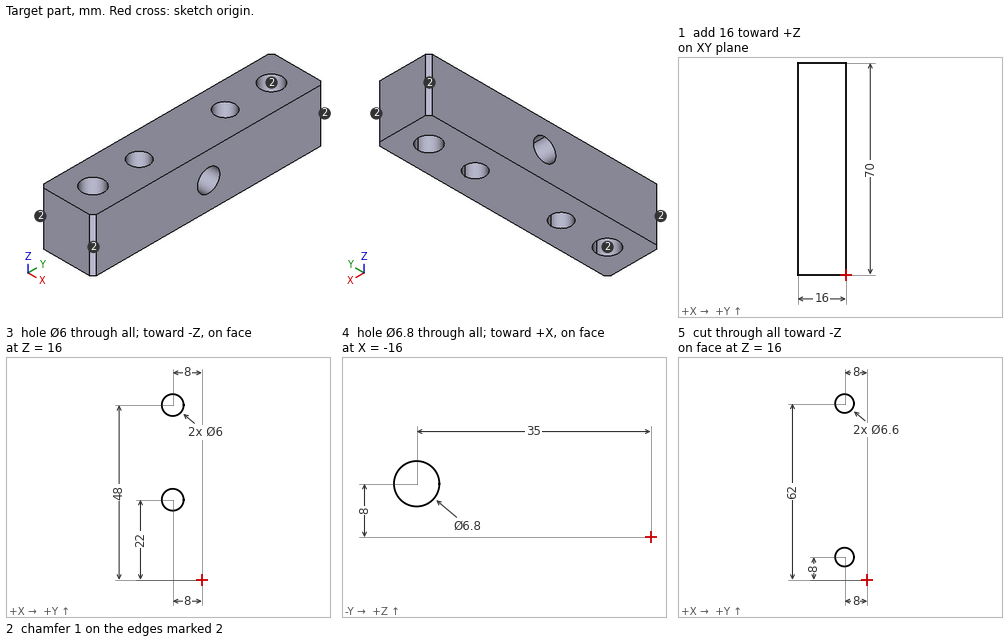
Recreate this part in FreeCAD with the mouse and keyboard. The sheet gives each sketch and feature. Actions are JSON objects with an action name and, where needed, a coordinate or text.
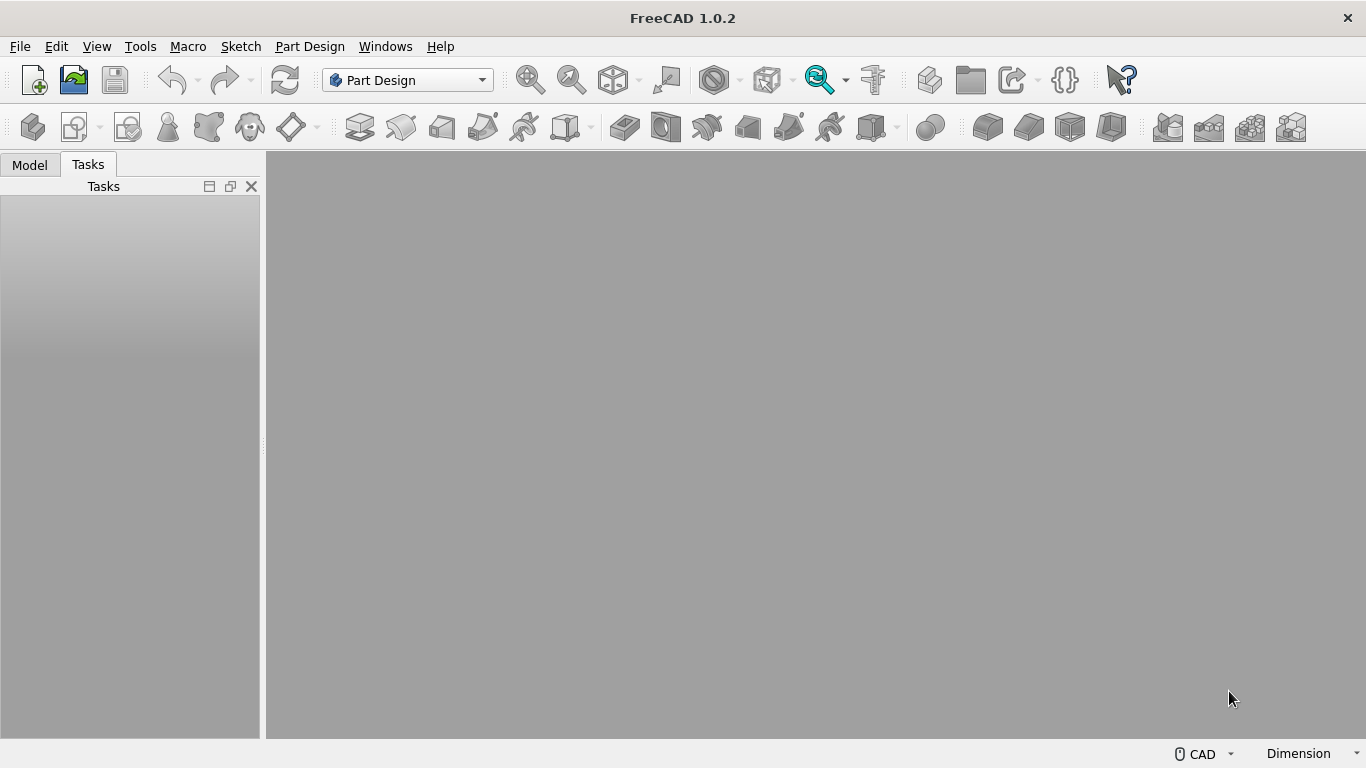
{"action": "key", "text": "ctrl+n"}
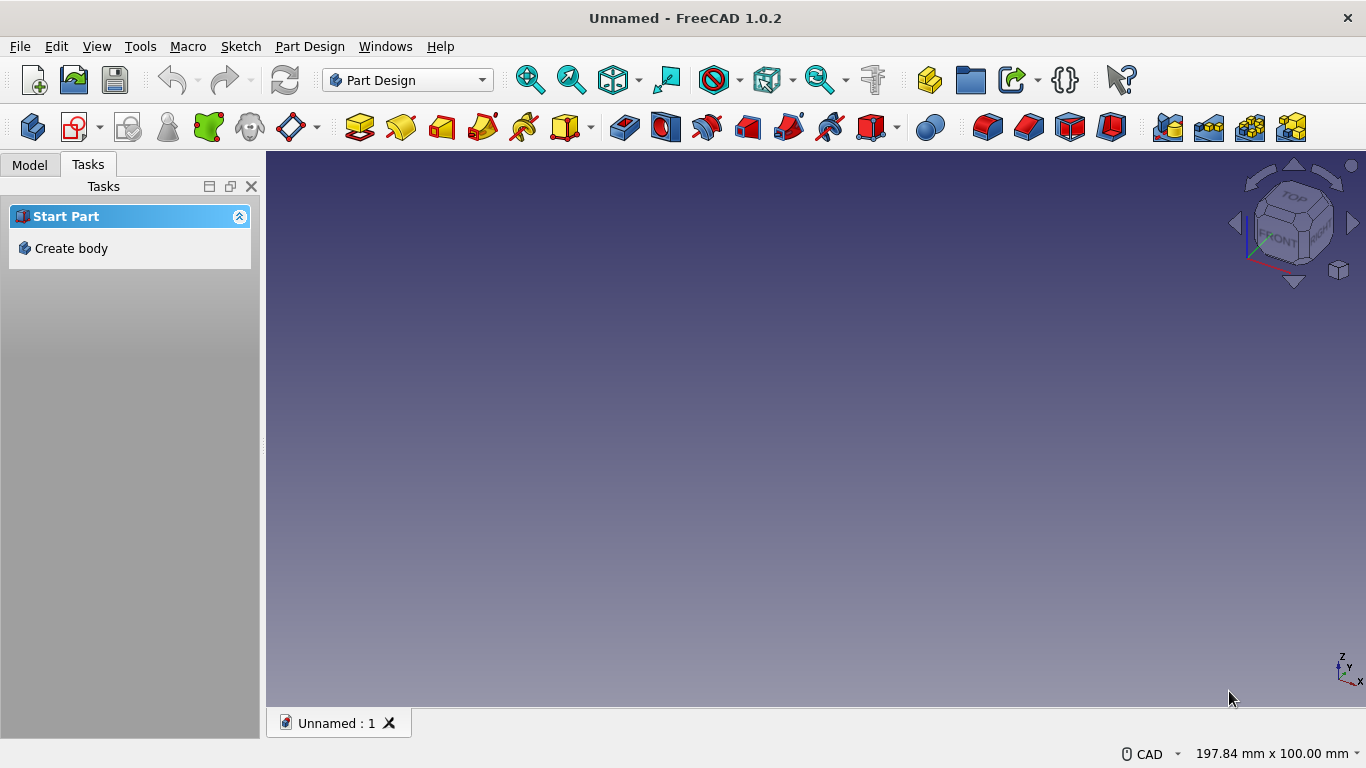
{"action": "left_click", "coordinate": [74, 128]}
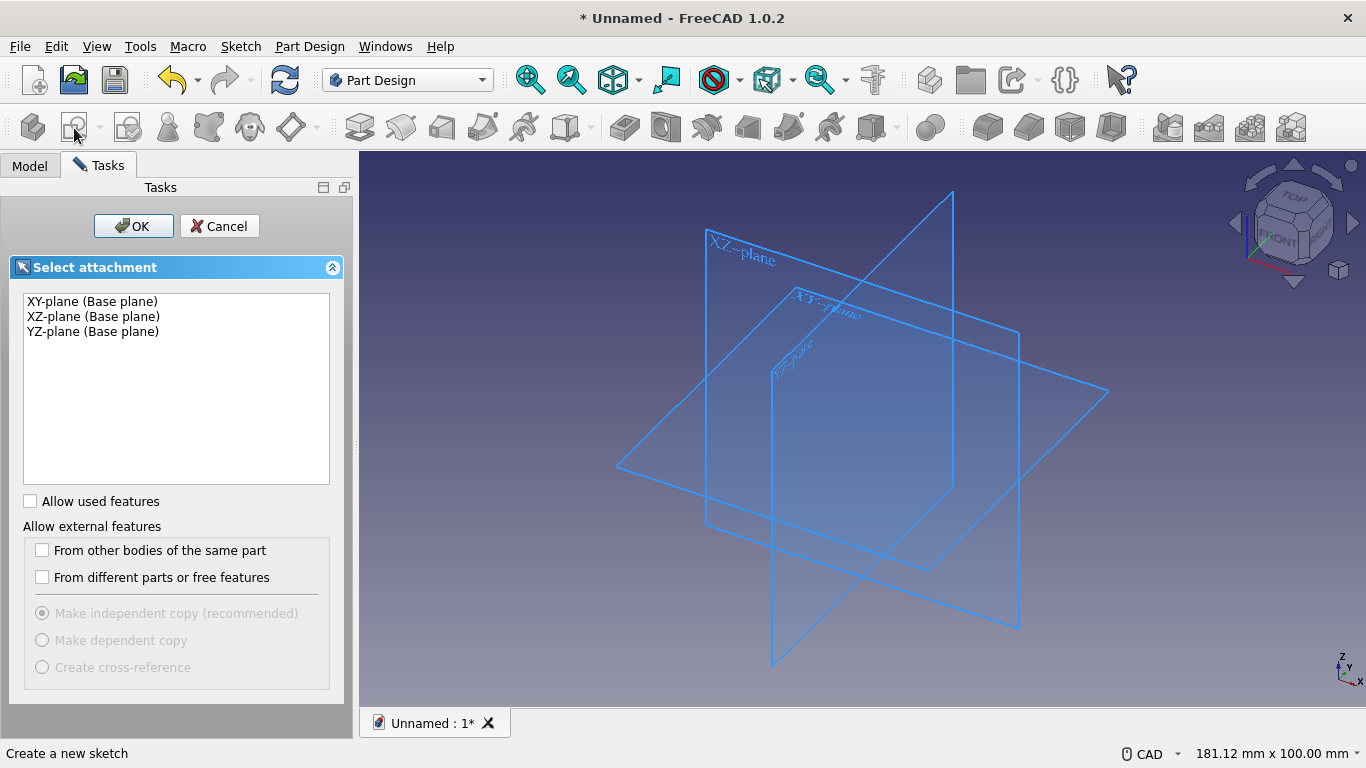
{"action": "left_click", "coordinate": [84, 302]}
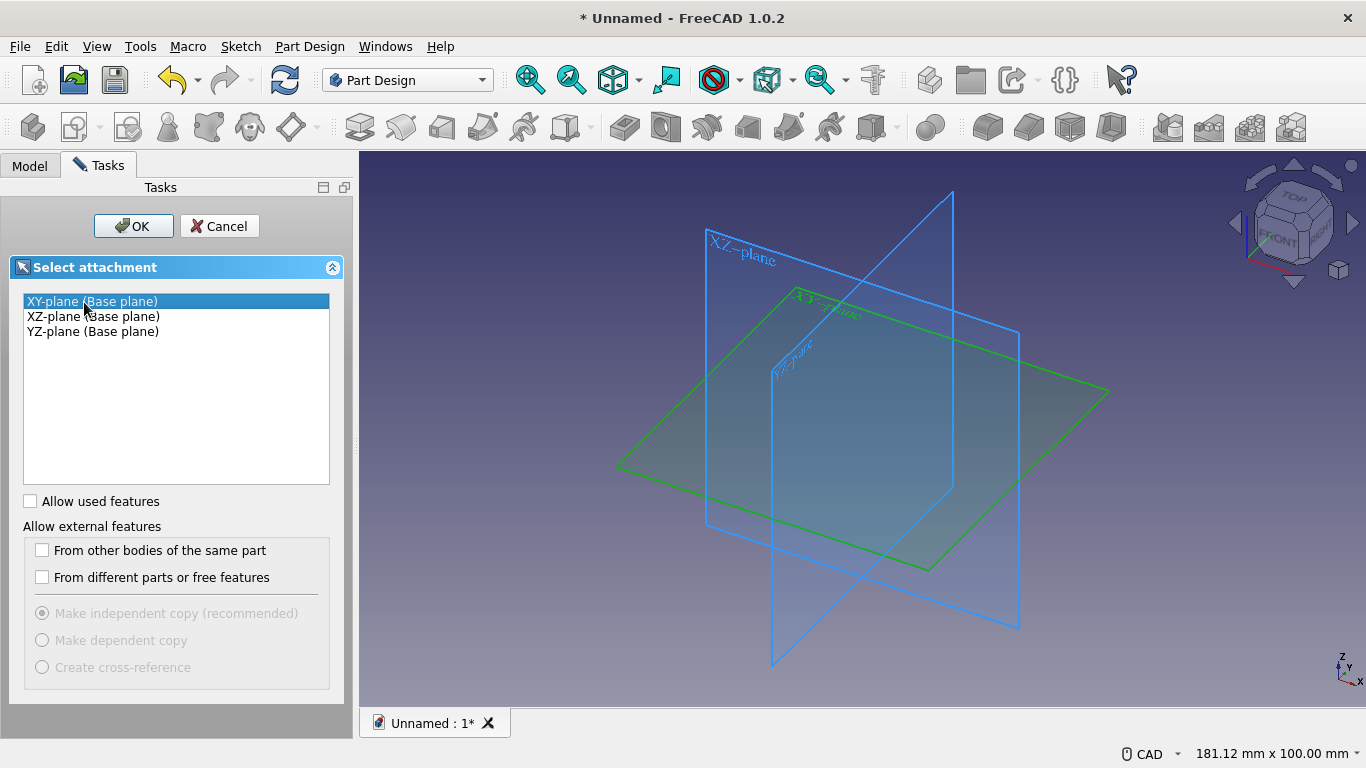
{"action": "left_click", "coordinate": [134, 226]}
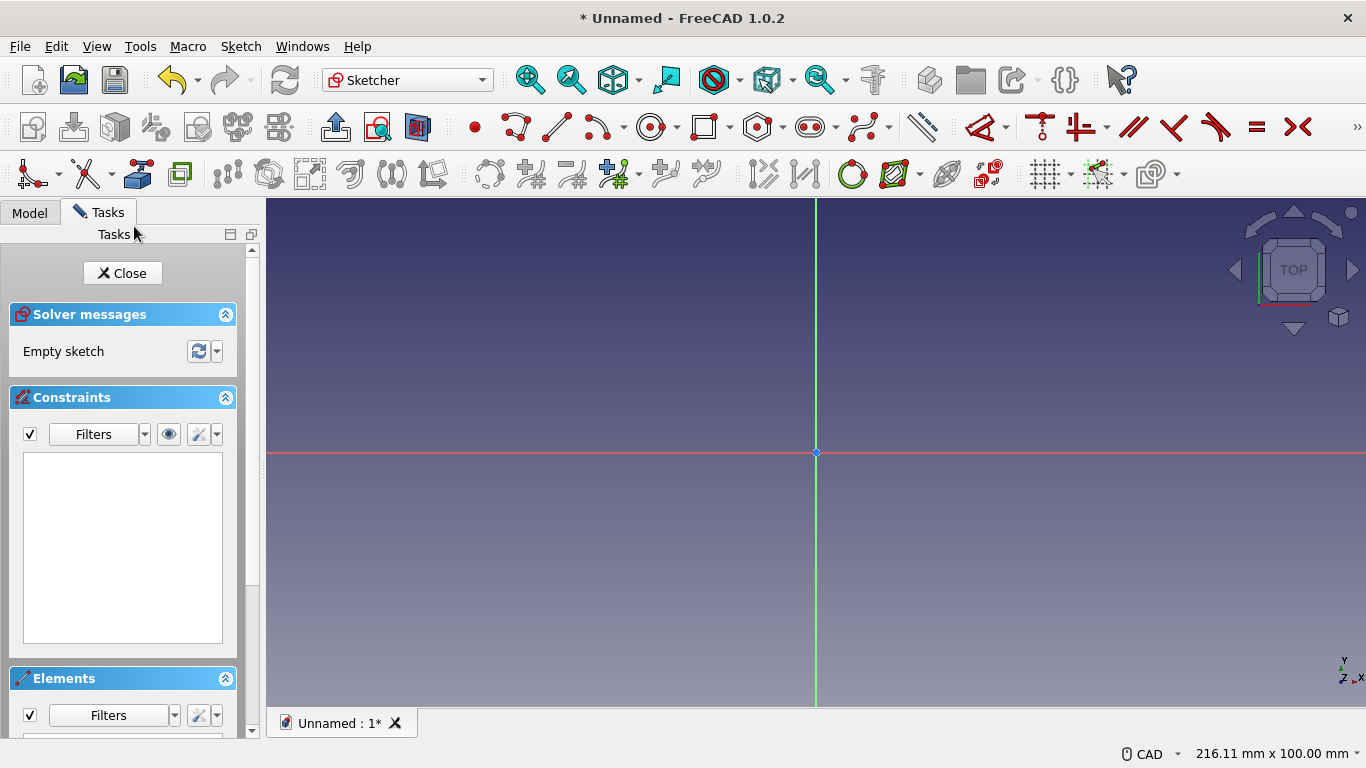
{"action": "scroll", "coordinate": [691, 679], "scroll_direction": "down", "scroll_amount": 2}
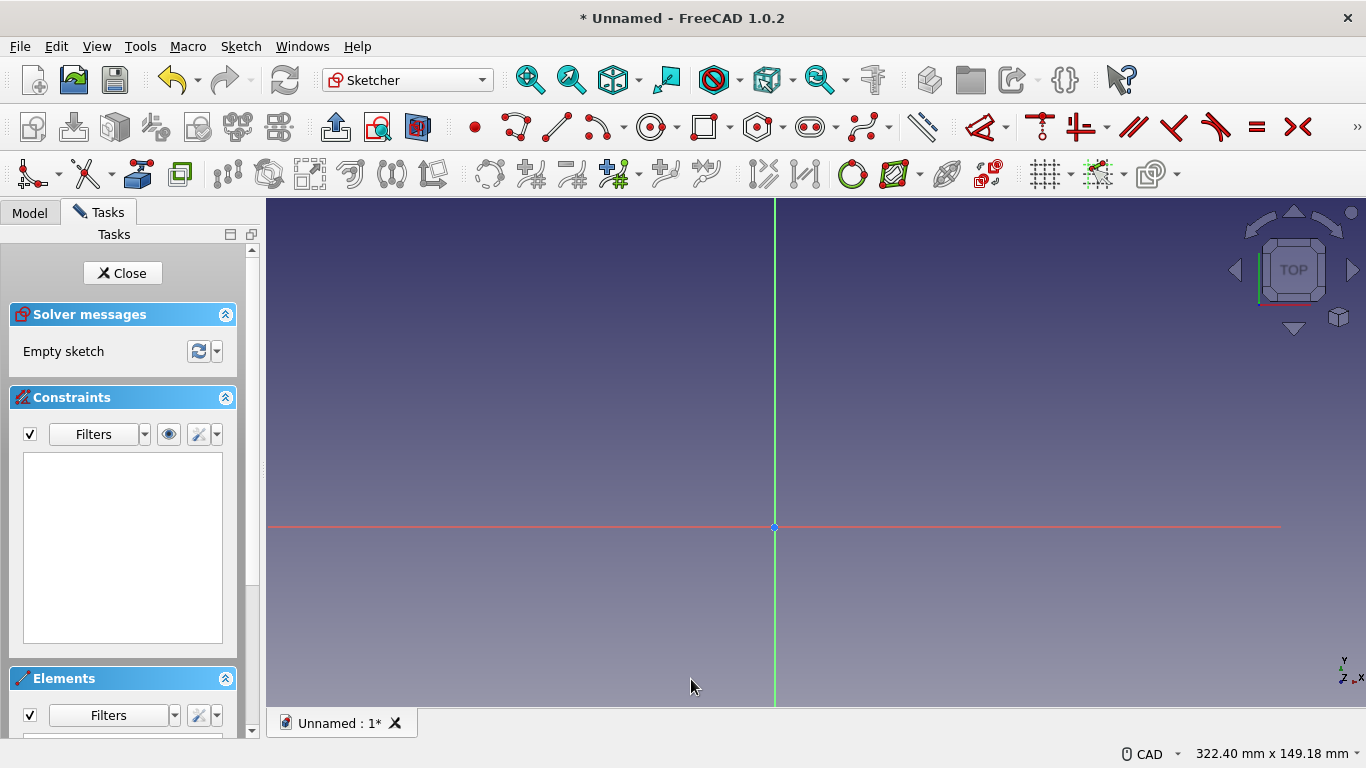
{"action": "left_click", "coordinate": [704, 128]}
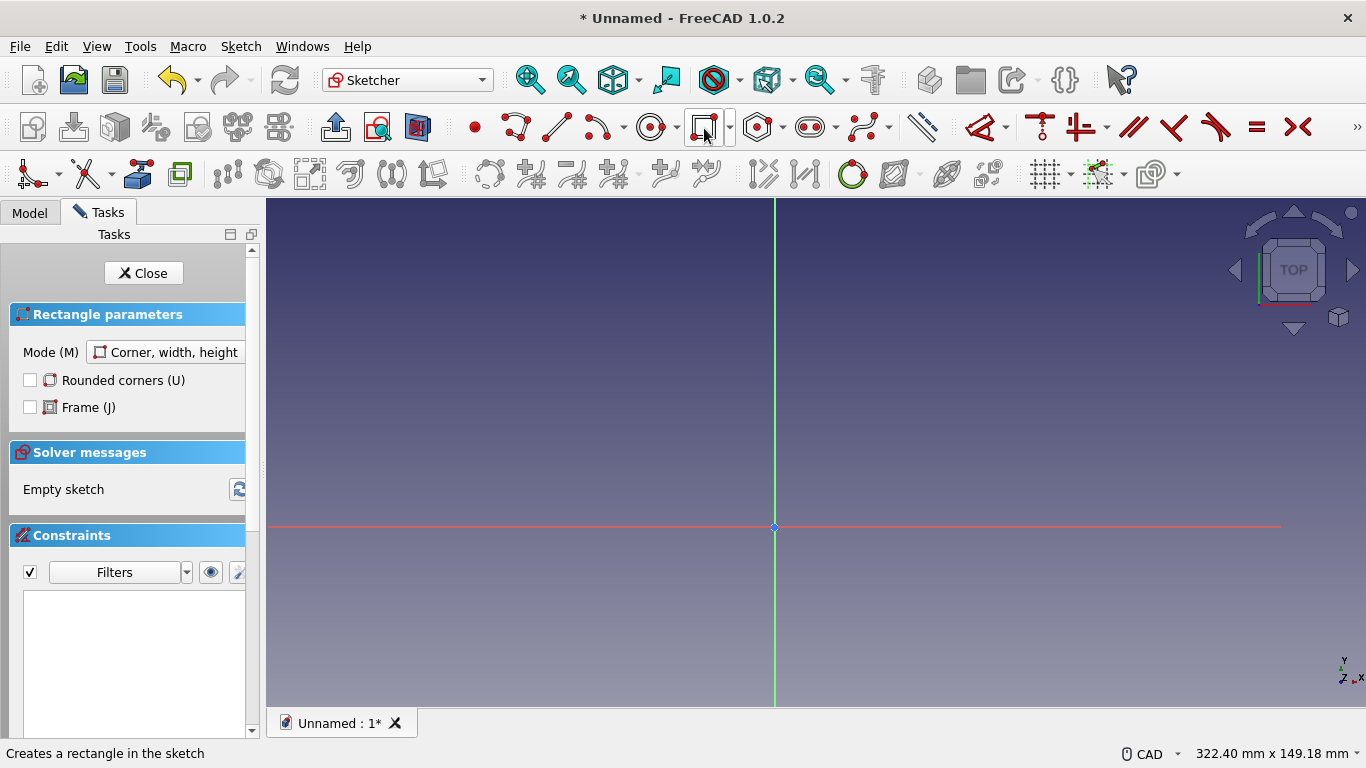
{"action": "left_click", "coordinate": [775, 527]}
{"action": "mouse_move", "coordinate": [720, 289]}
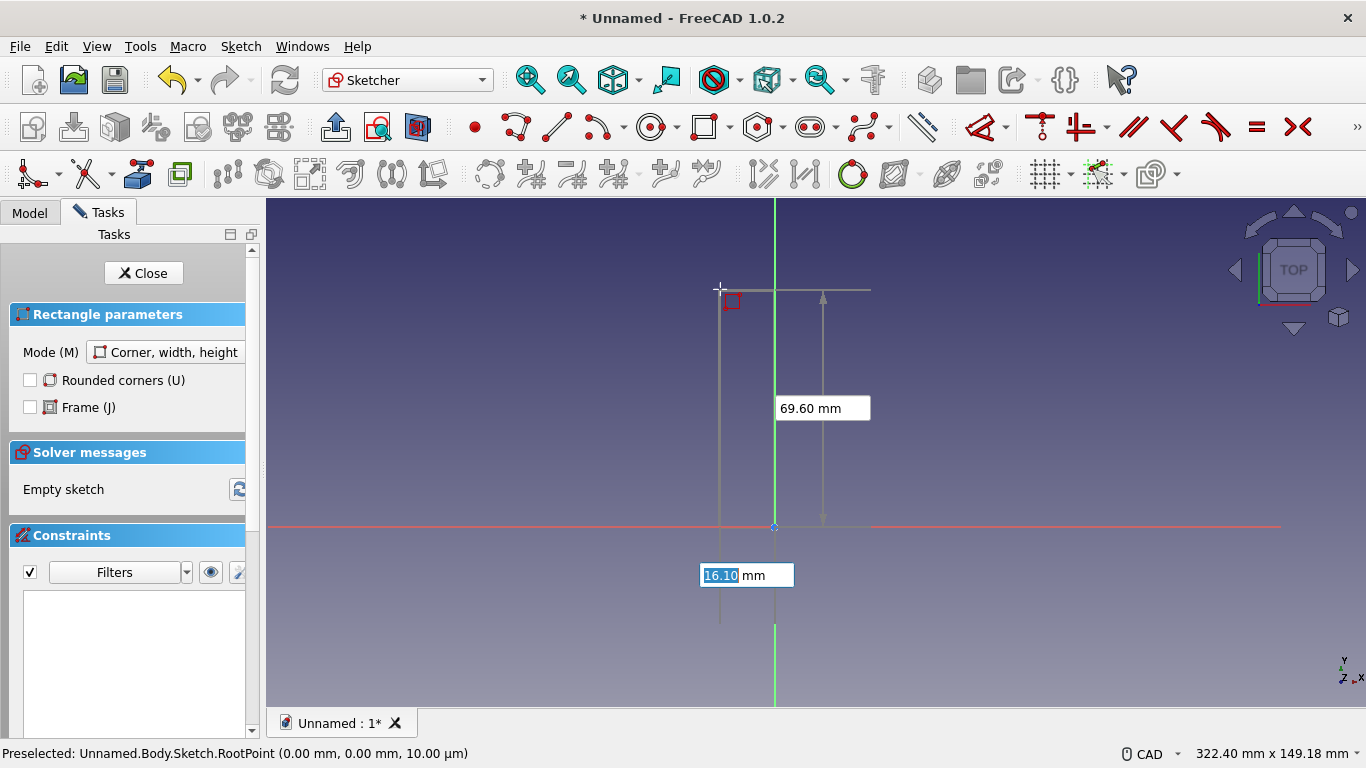
{"action": "type", "text": "16"}
{"action": "key", "text": "Tab"}
{"action": "type", "text": "70"}
{"action": "key", "text": "Return"}
{"action": "key", "text": "Escape"}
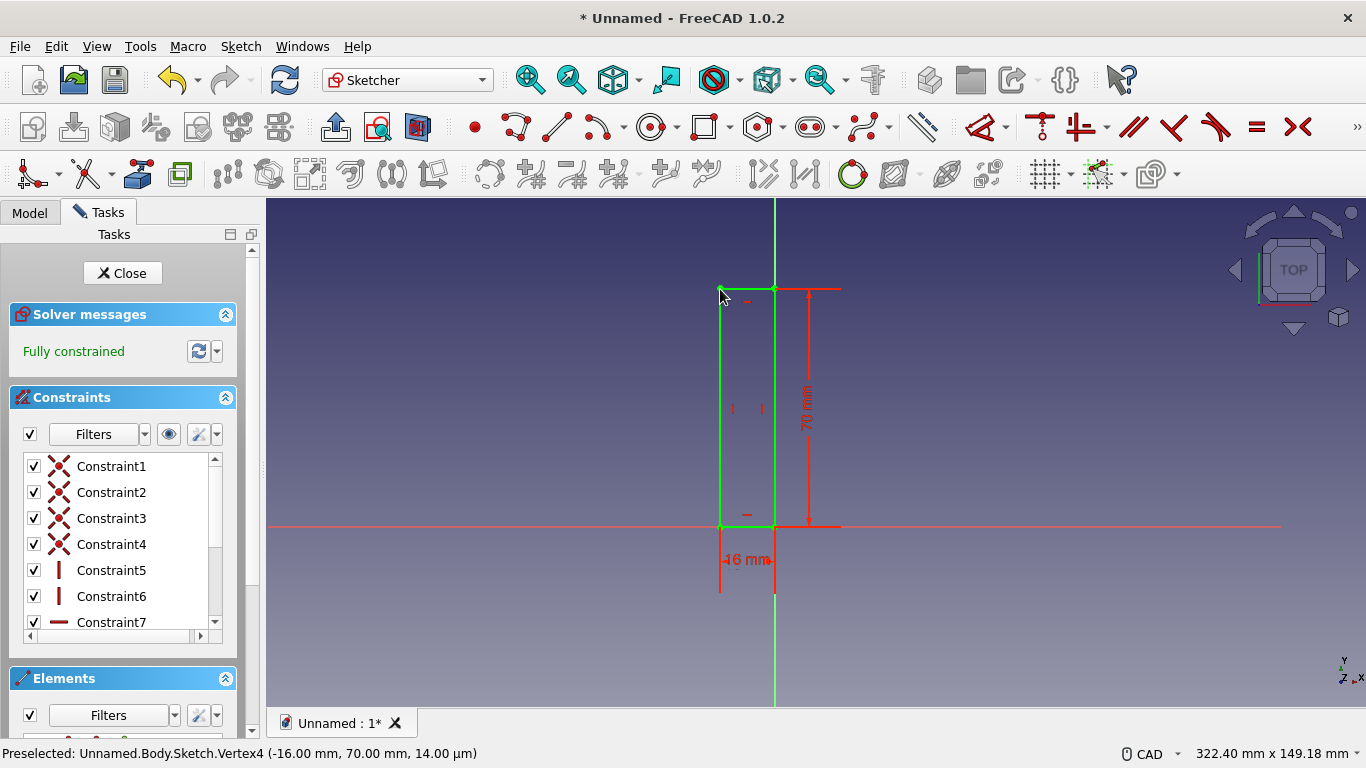
{"action": "left_click", "coordinate": [123, 273]}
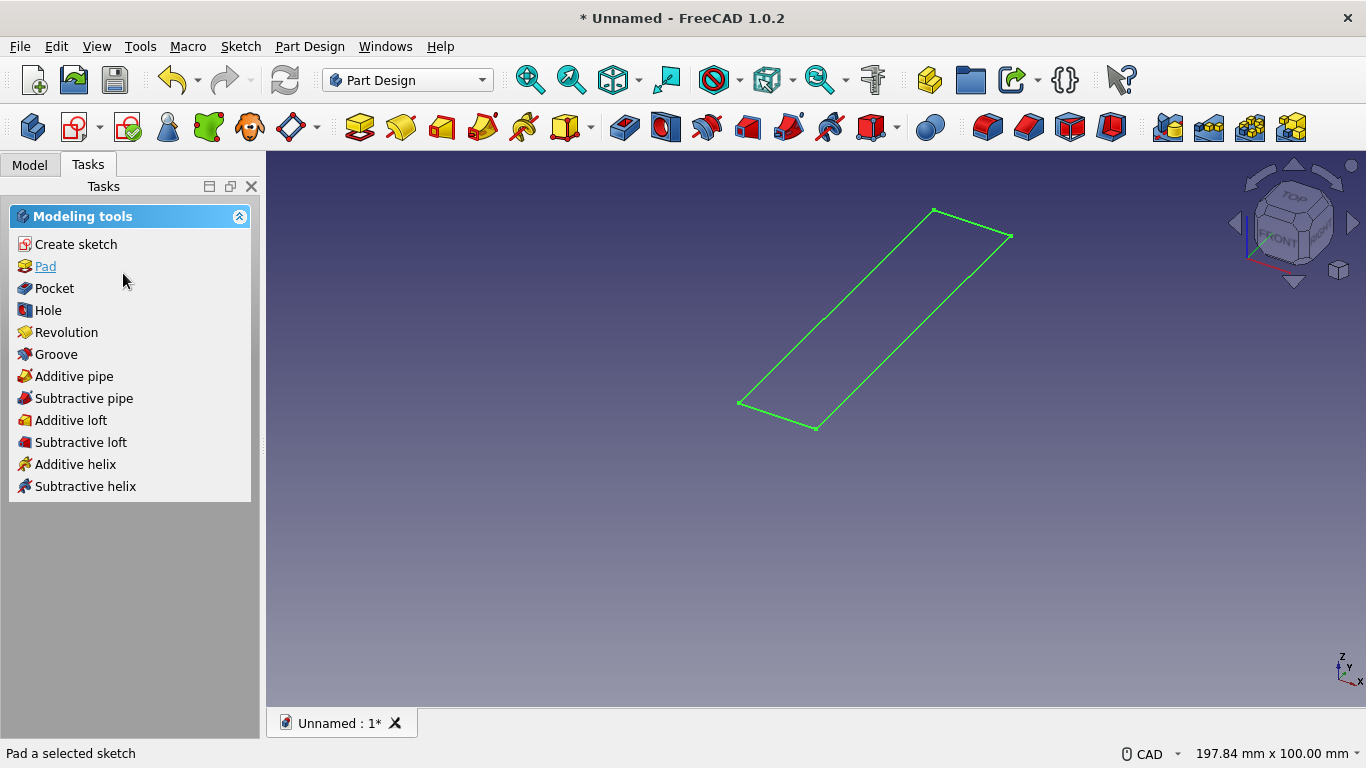
{"action": "left_click", "coordinate": [360, 128]}